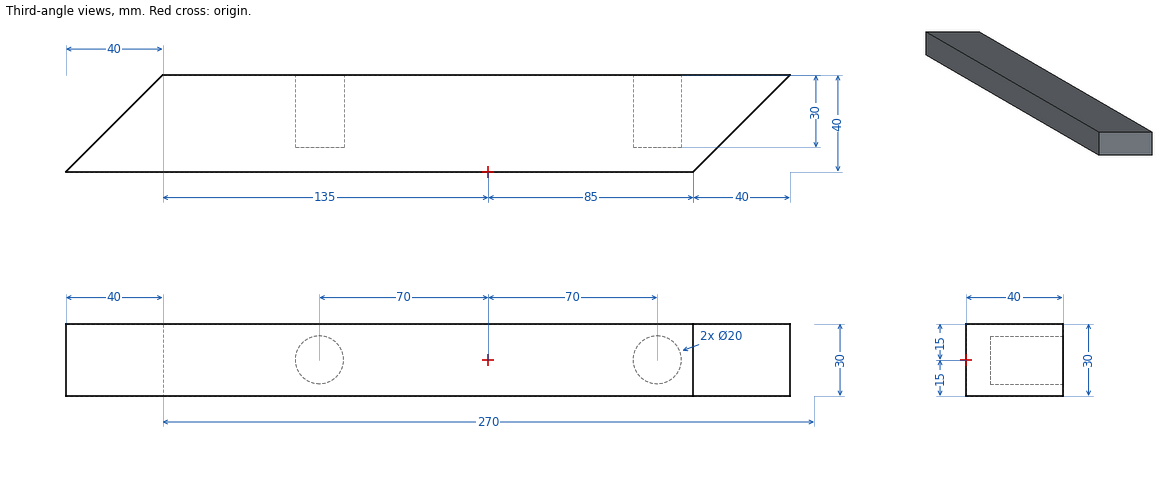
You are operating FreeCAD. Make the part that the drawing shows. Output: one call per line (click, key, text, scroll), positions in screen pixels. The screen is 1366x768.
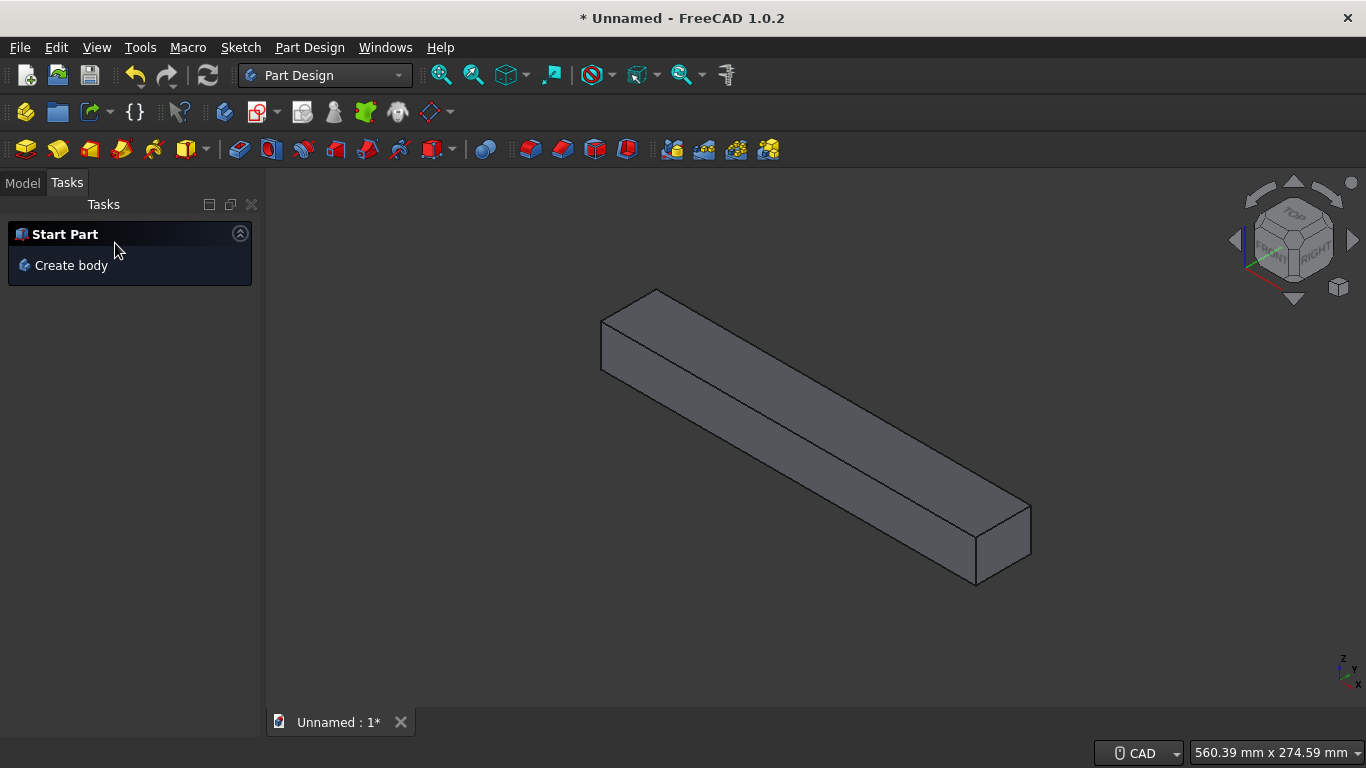
click(1003, 545)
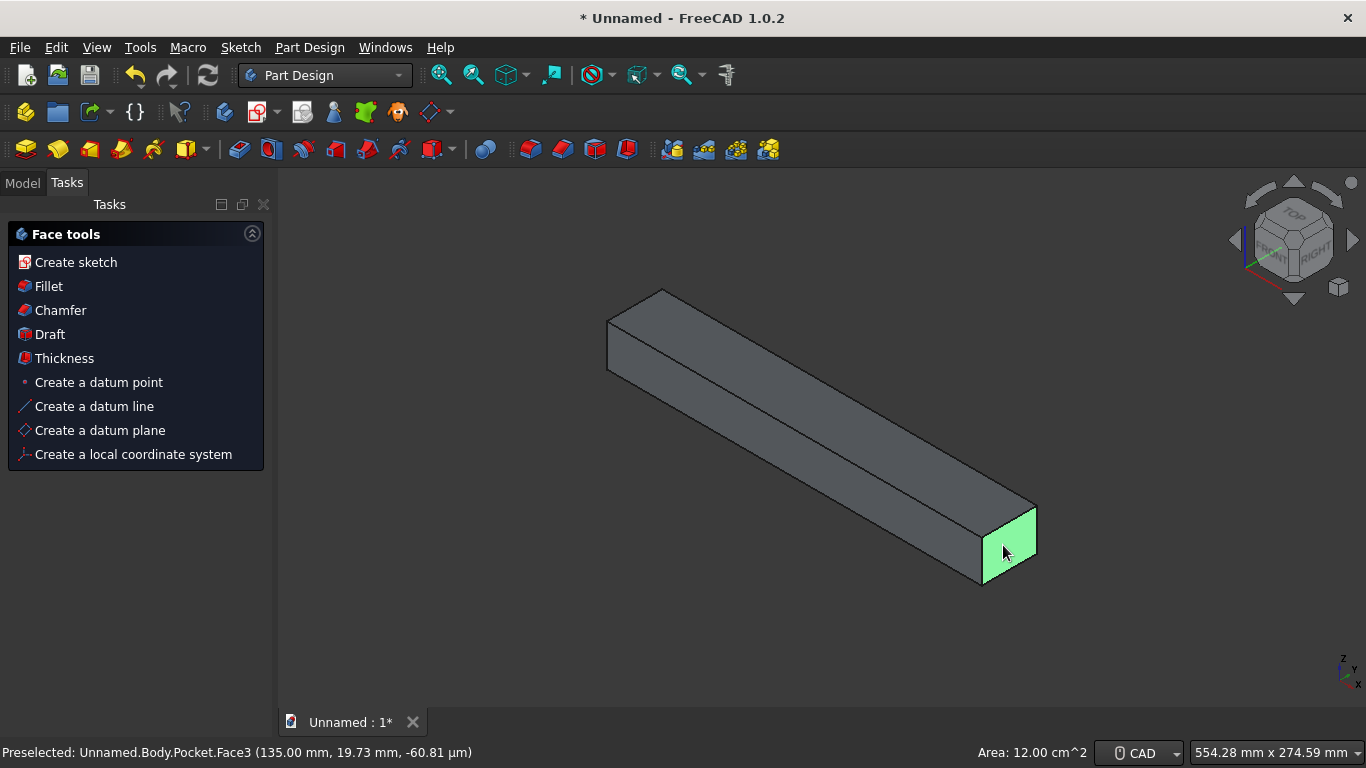
click(258, 112)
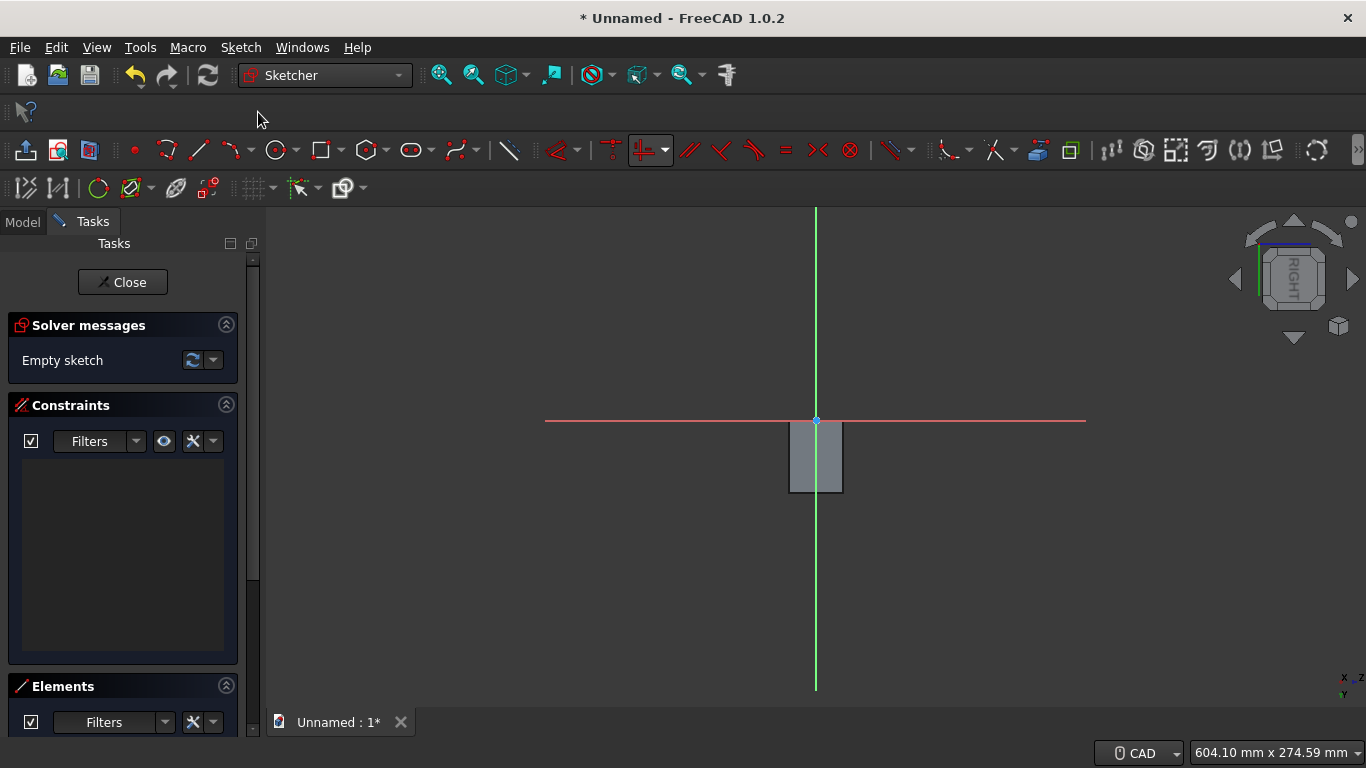
scroll(838, 457, up, 7)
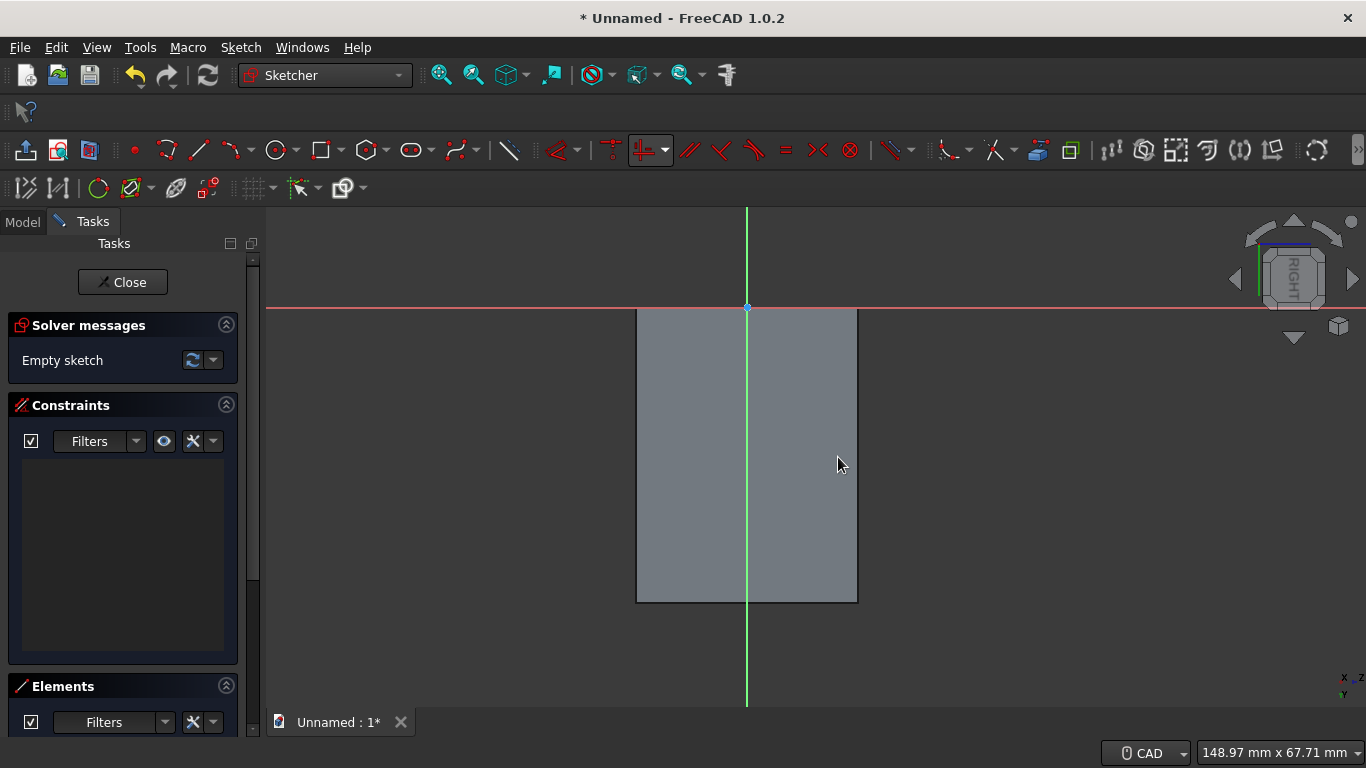
click(322, 150)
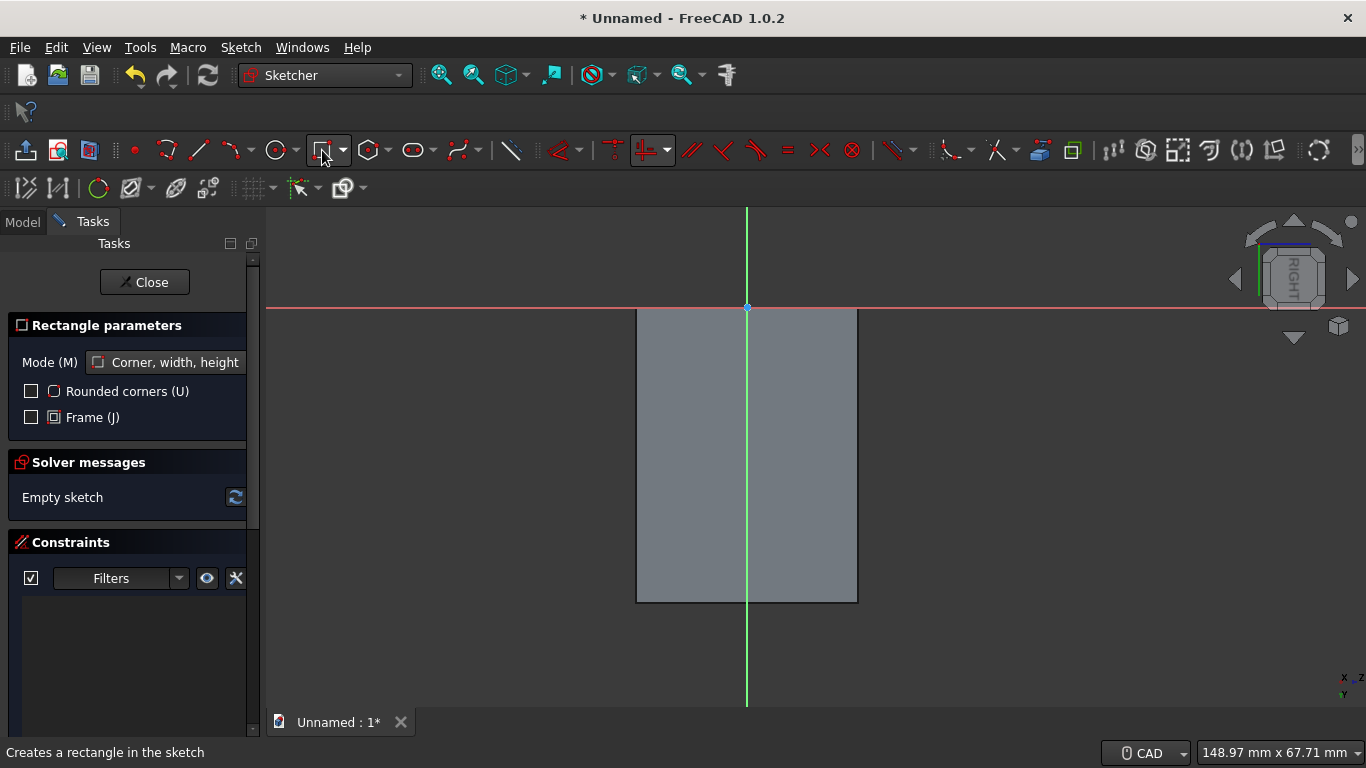
click(636, 308)
click(858, 603)
key(Escape)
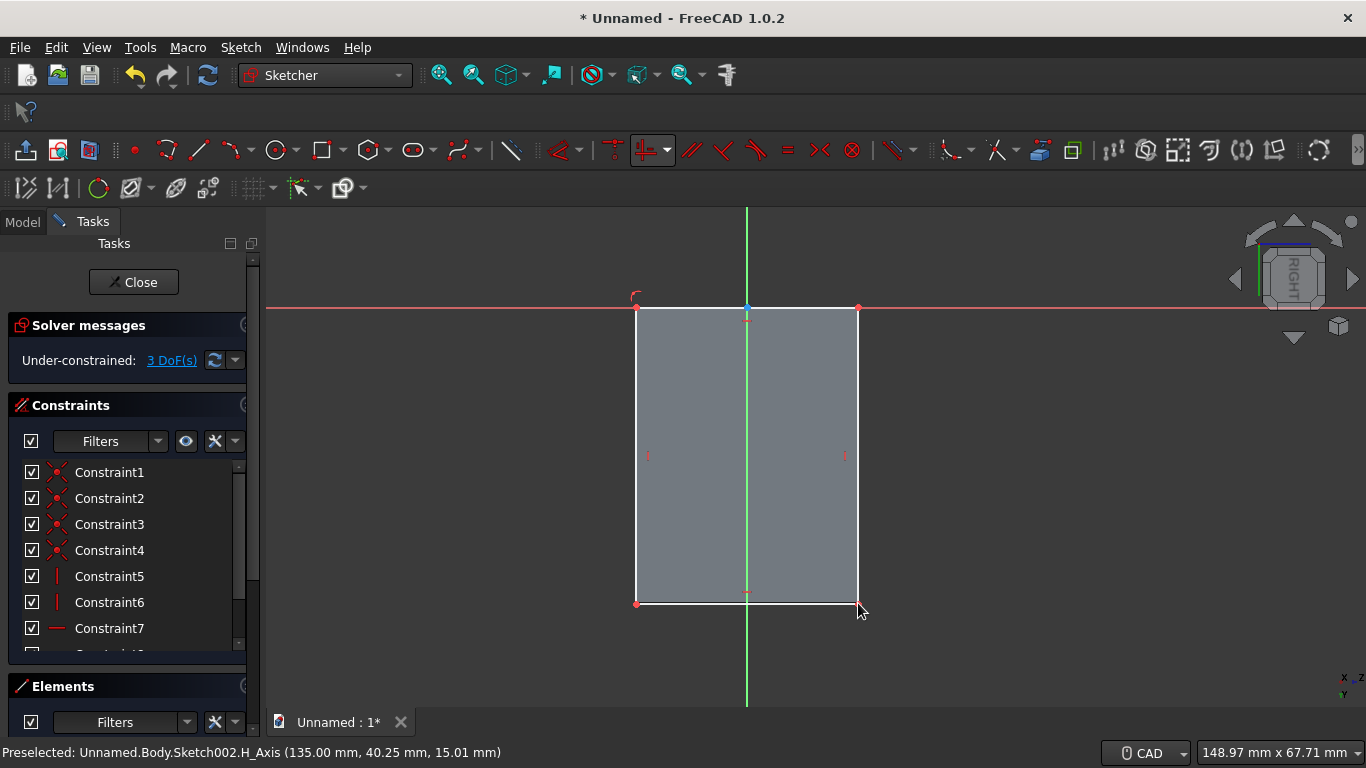
click(558, 150)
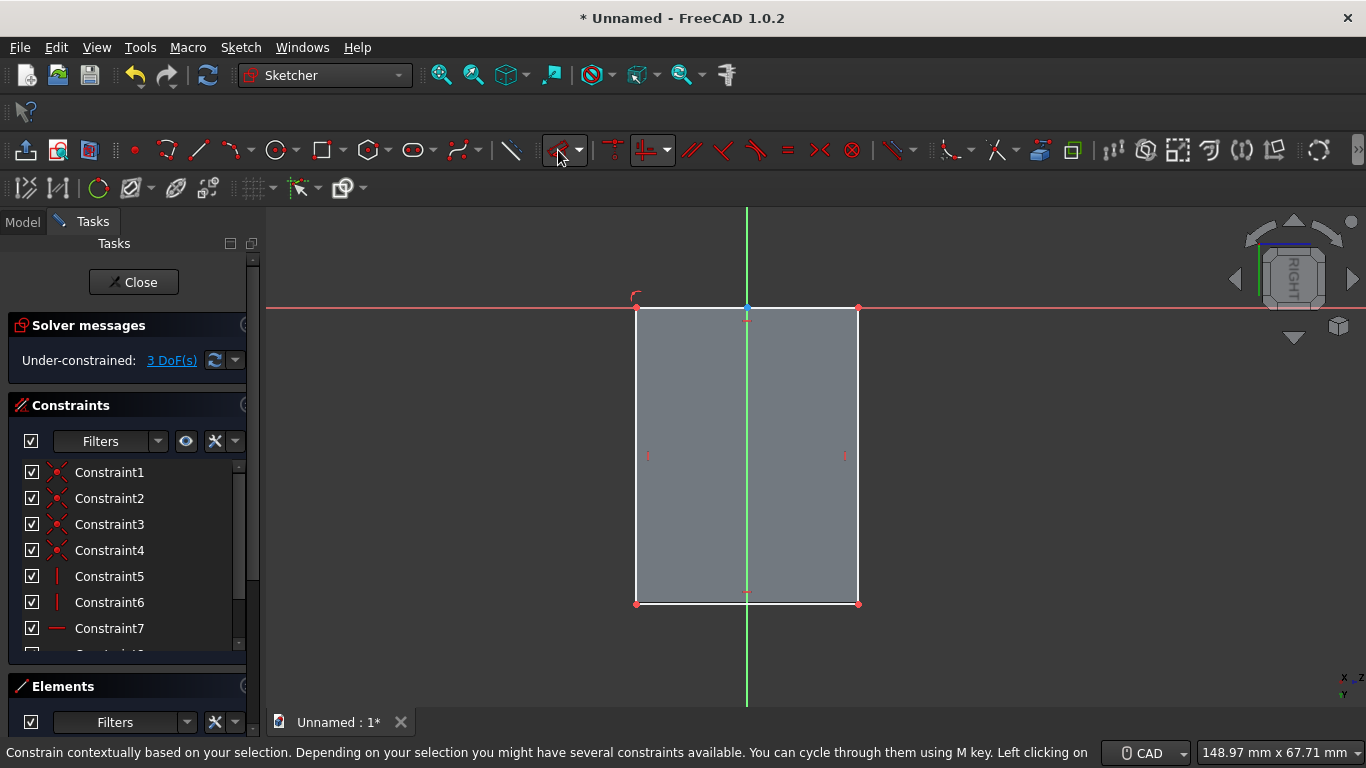
click(636, 397)
click(602, 456)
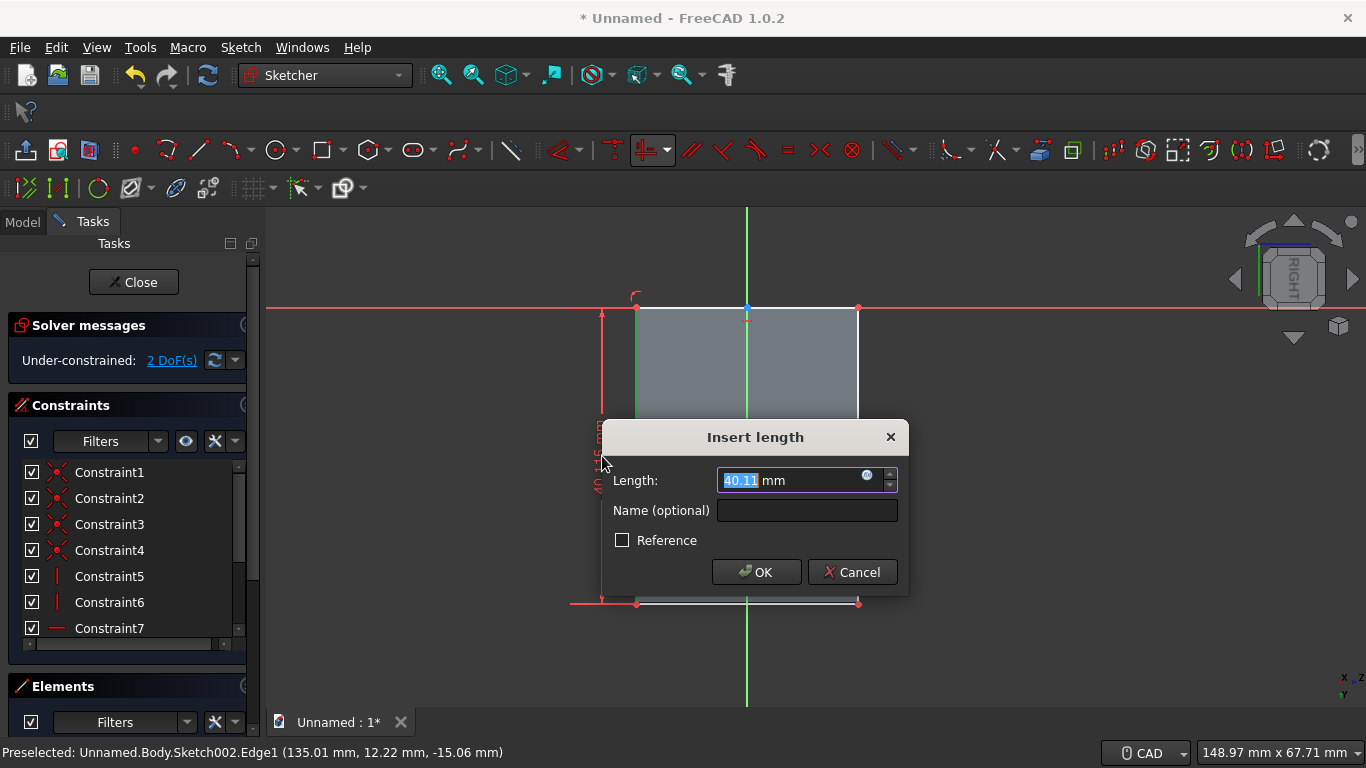
text(40)
key(Return)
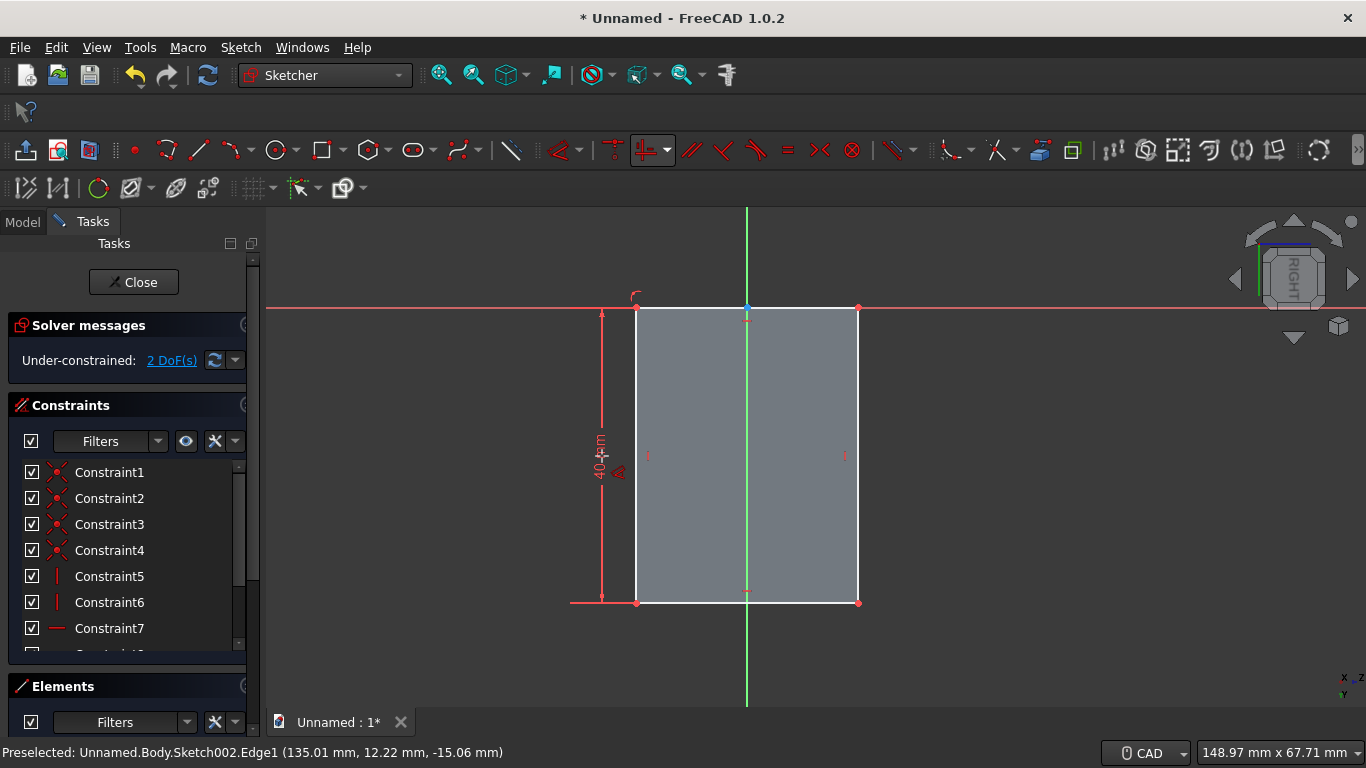
click(703, 603)
click(696, 637)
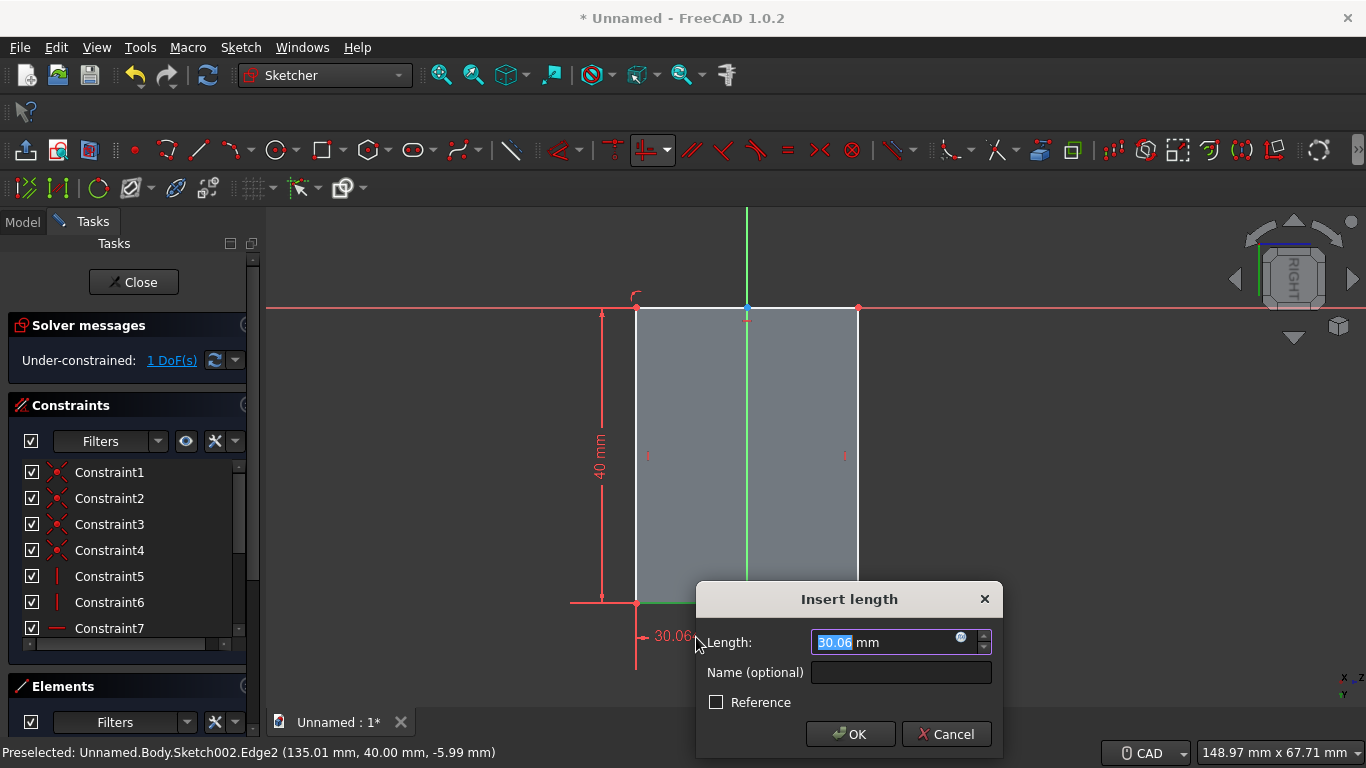
text(30)
key(Return)